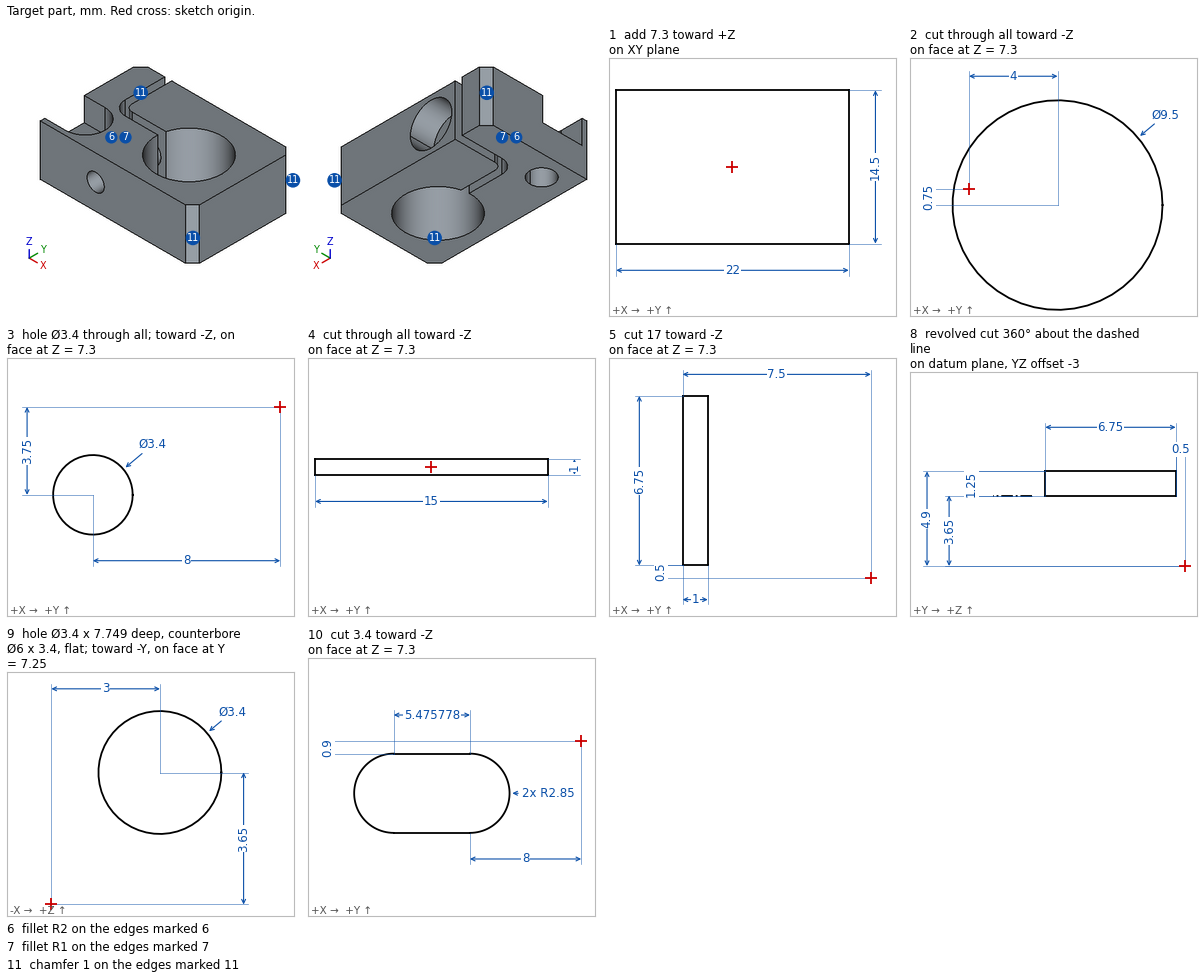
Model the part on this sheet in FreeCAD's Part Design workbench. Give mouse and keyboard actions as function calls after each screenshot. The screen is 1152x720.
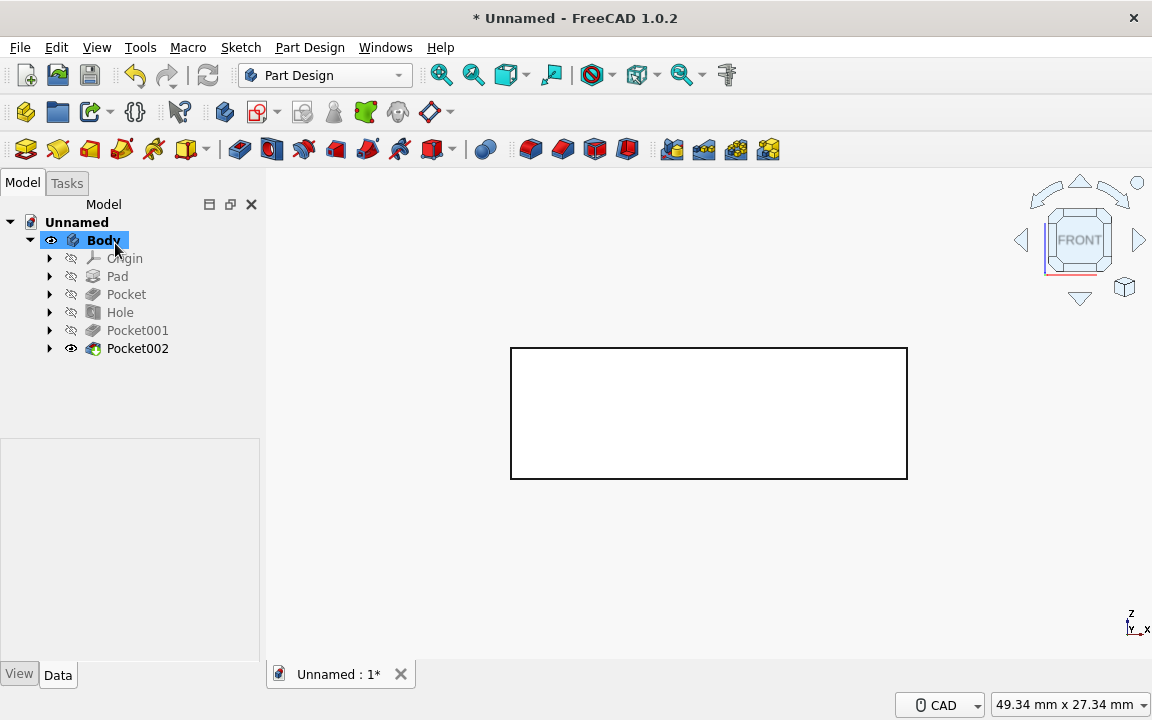
key(v)
key(f)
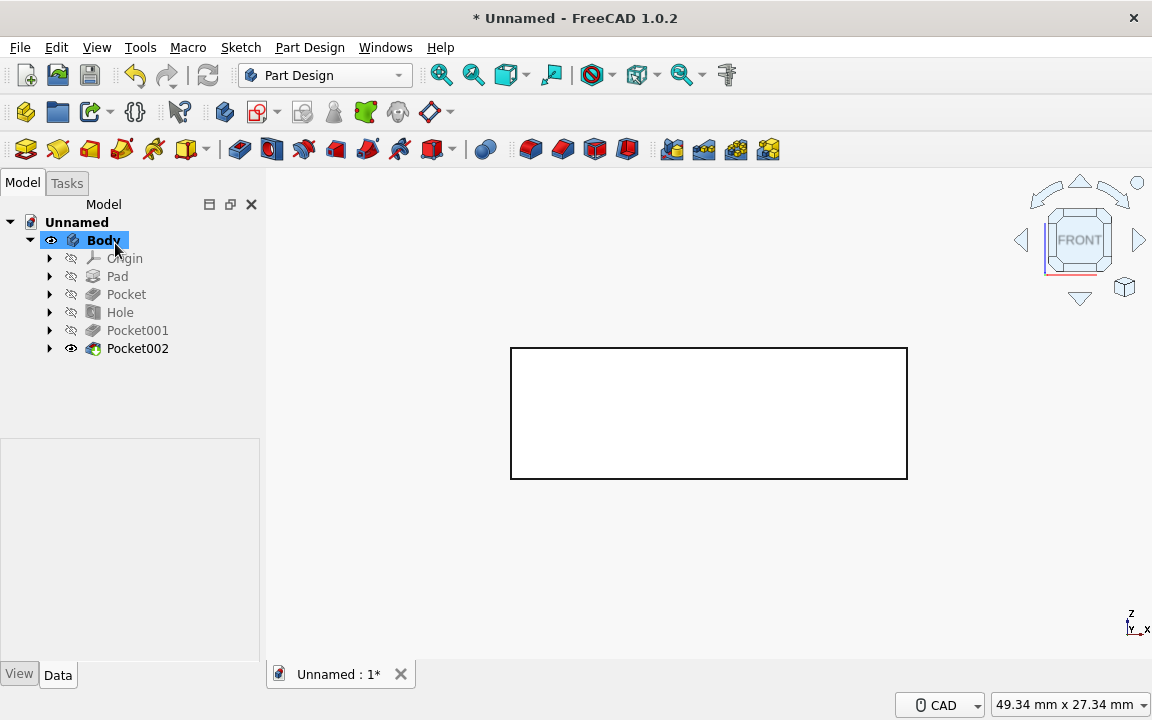
key(3)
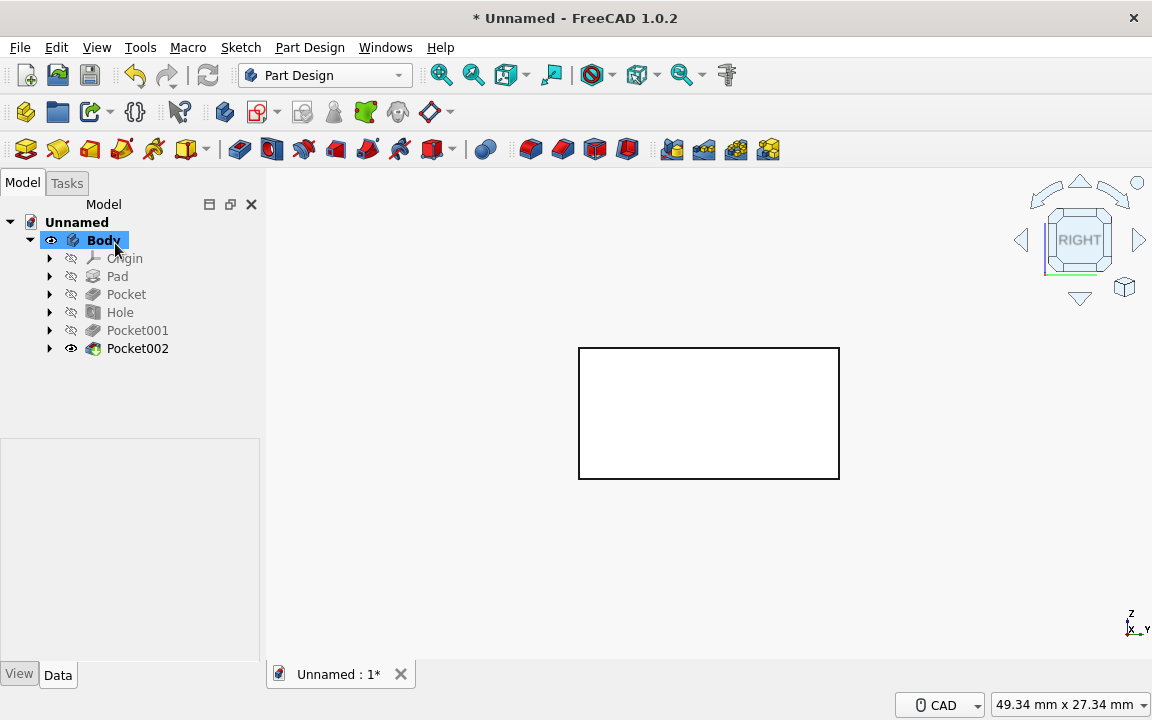
click(442, 76)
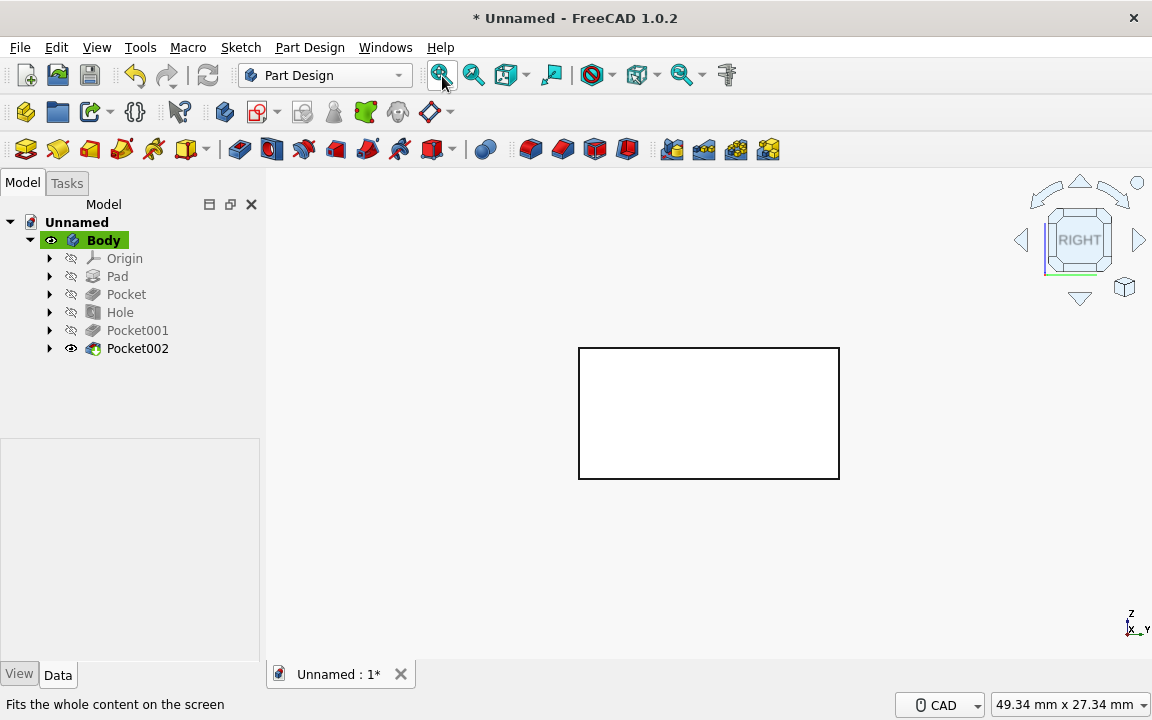
key(5)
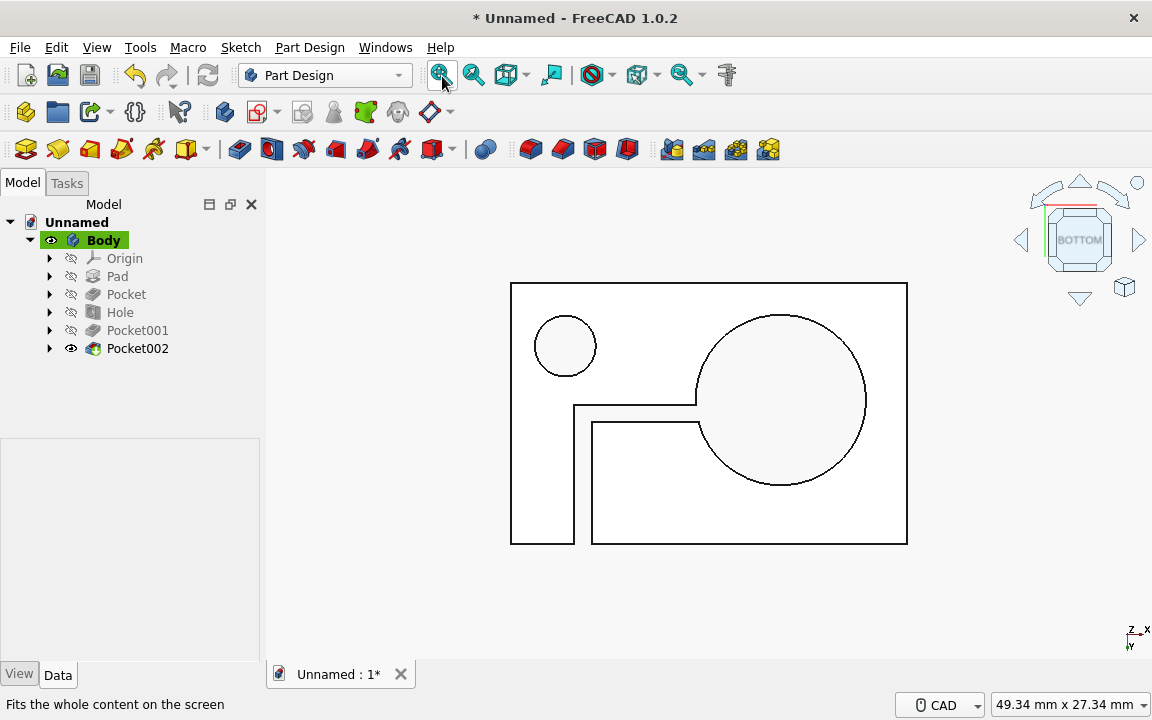
key(4)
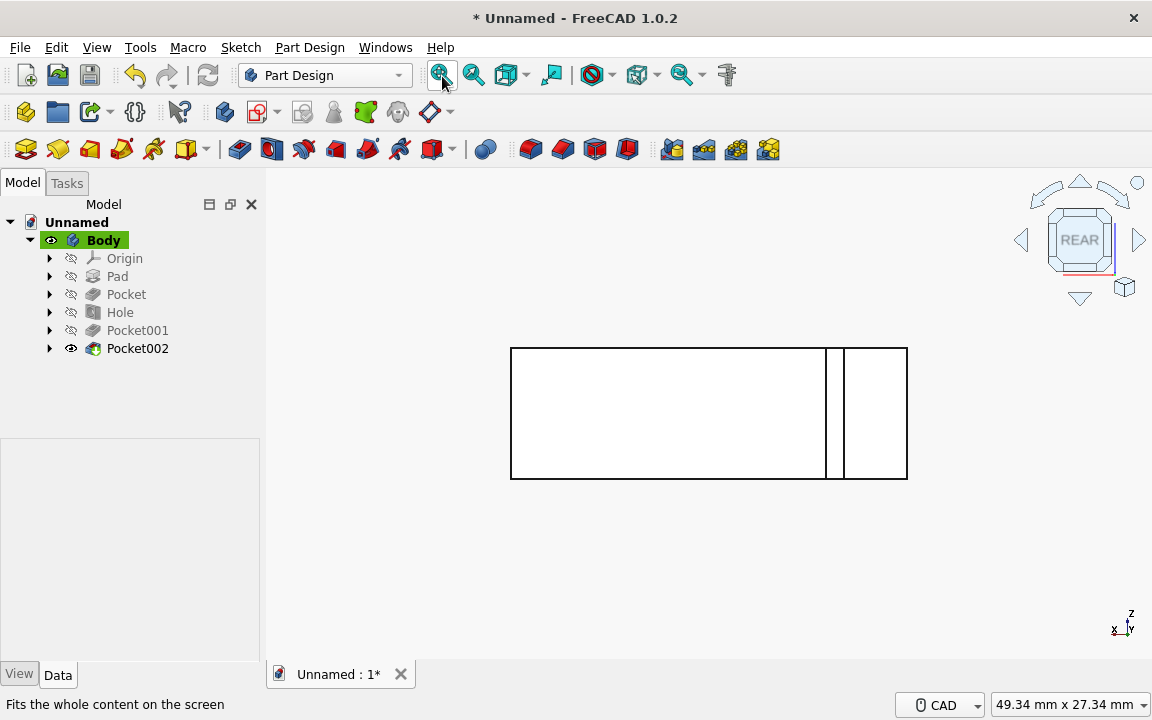
click(442, 76)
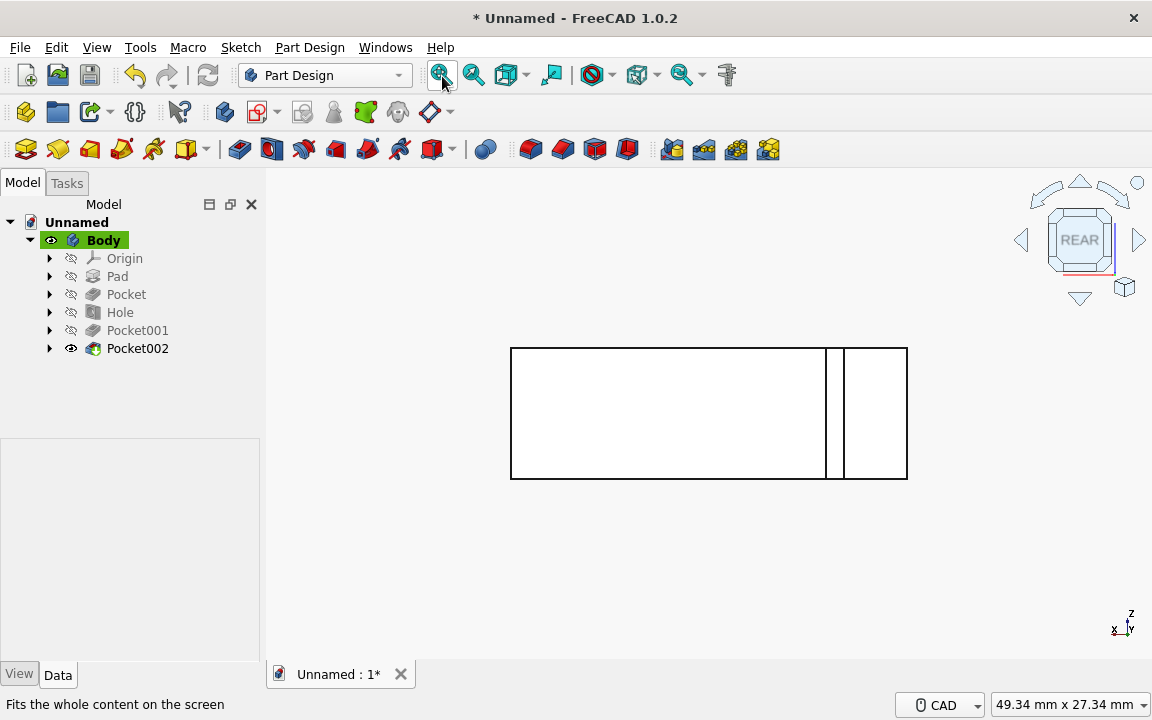
key(6)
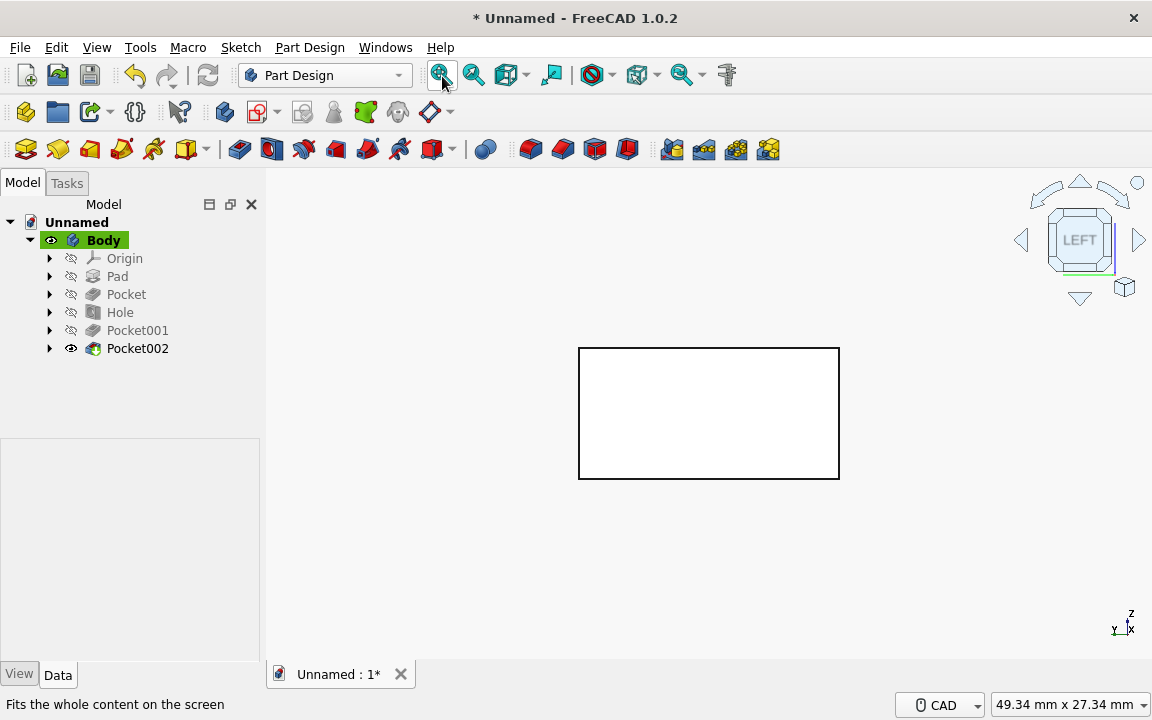
click(442, 76)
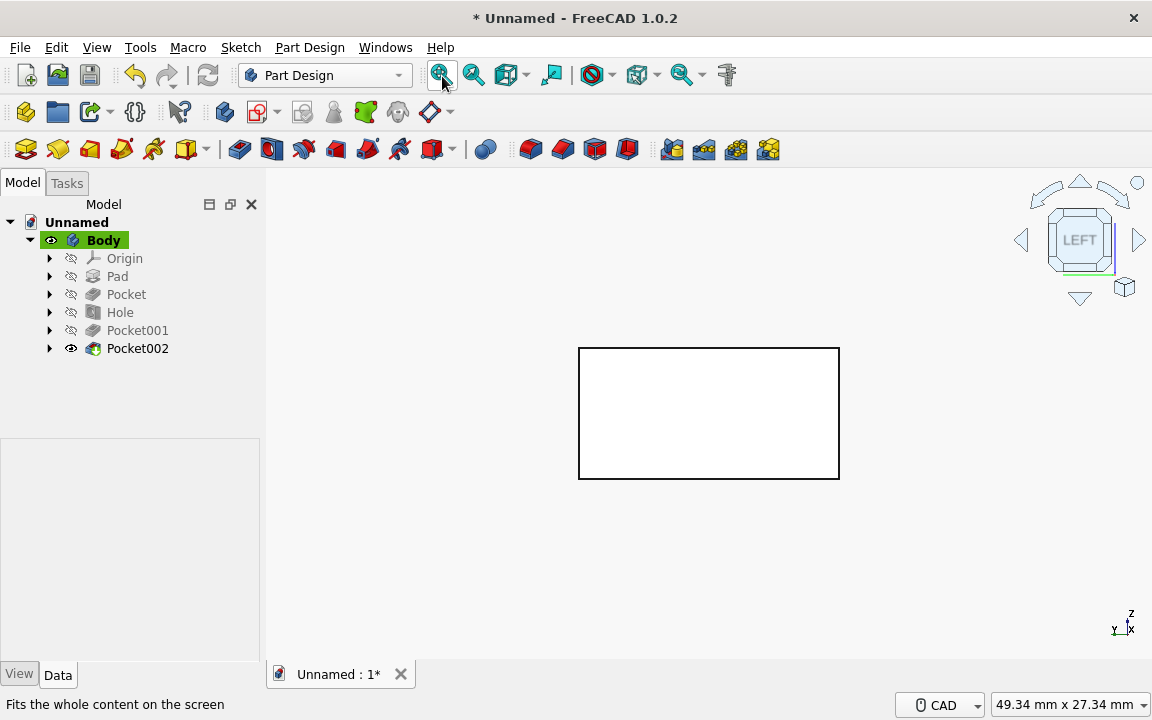
key(v)
key(3)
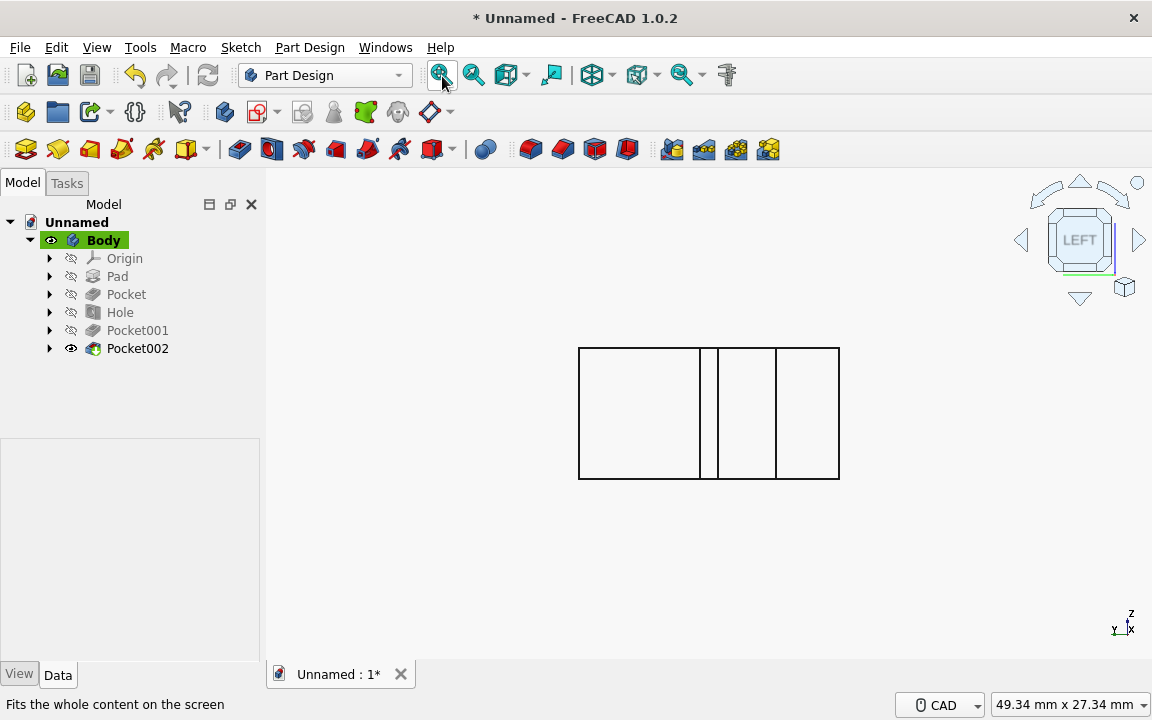
key(0)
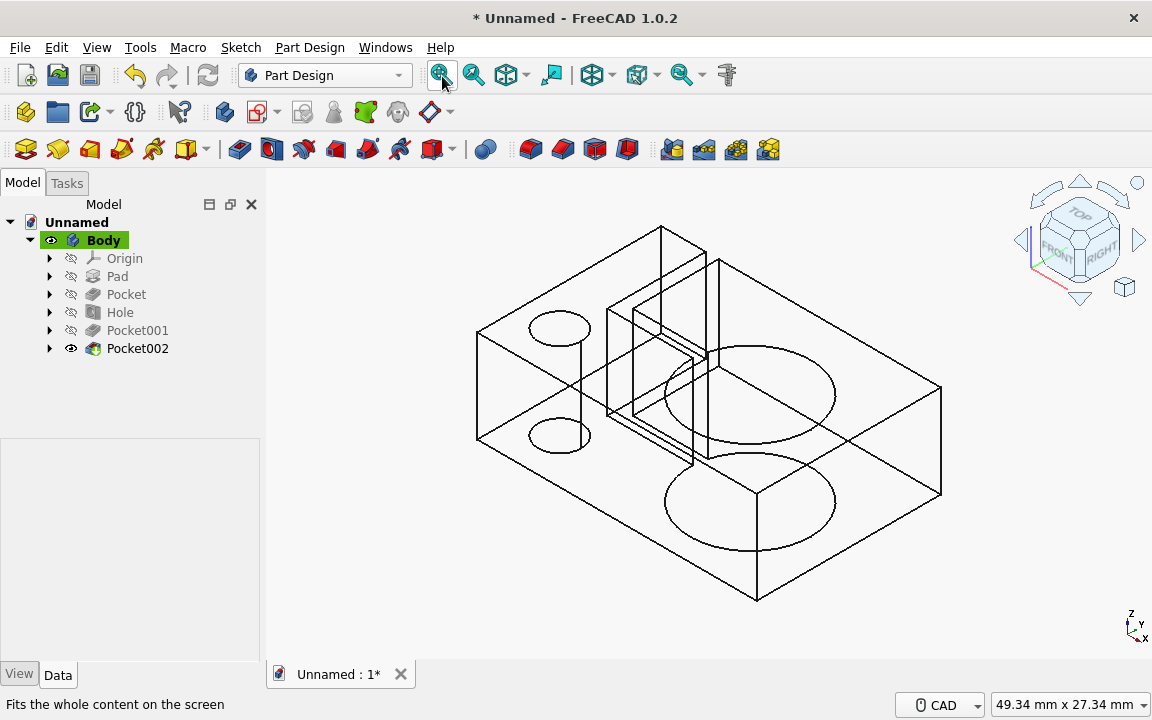
click(607, 361)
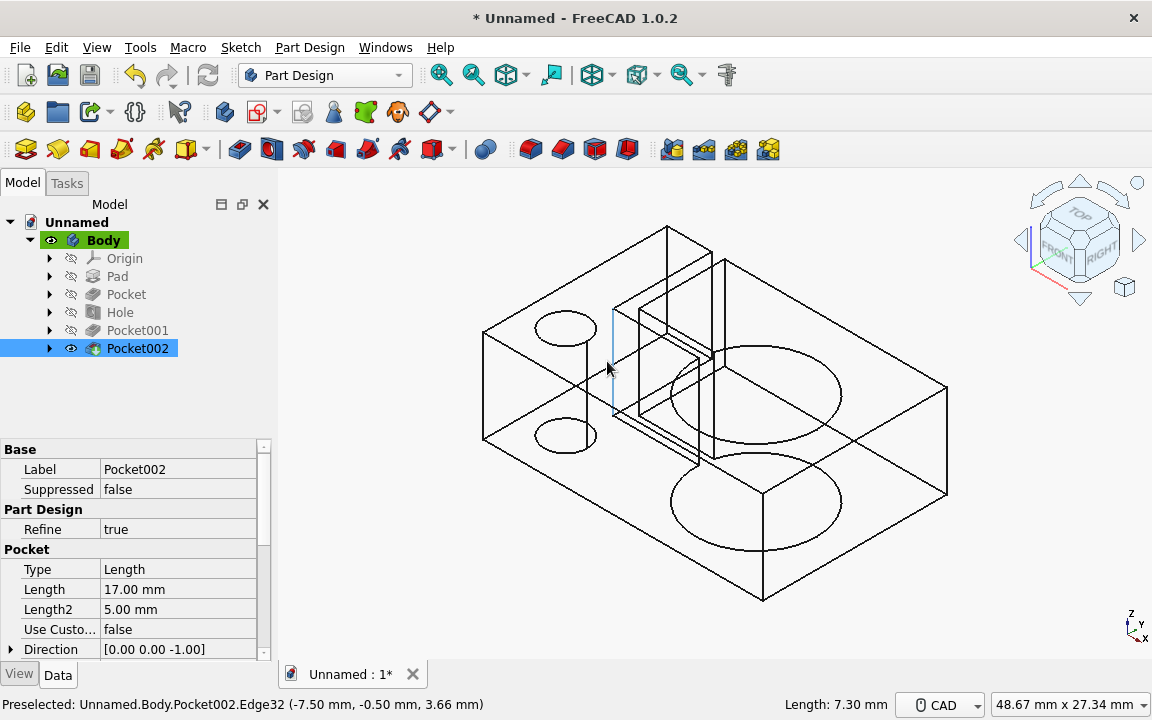
key(v)
key(1)